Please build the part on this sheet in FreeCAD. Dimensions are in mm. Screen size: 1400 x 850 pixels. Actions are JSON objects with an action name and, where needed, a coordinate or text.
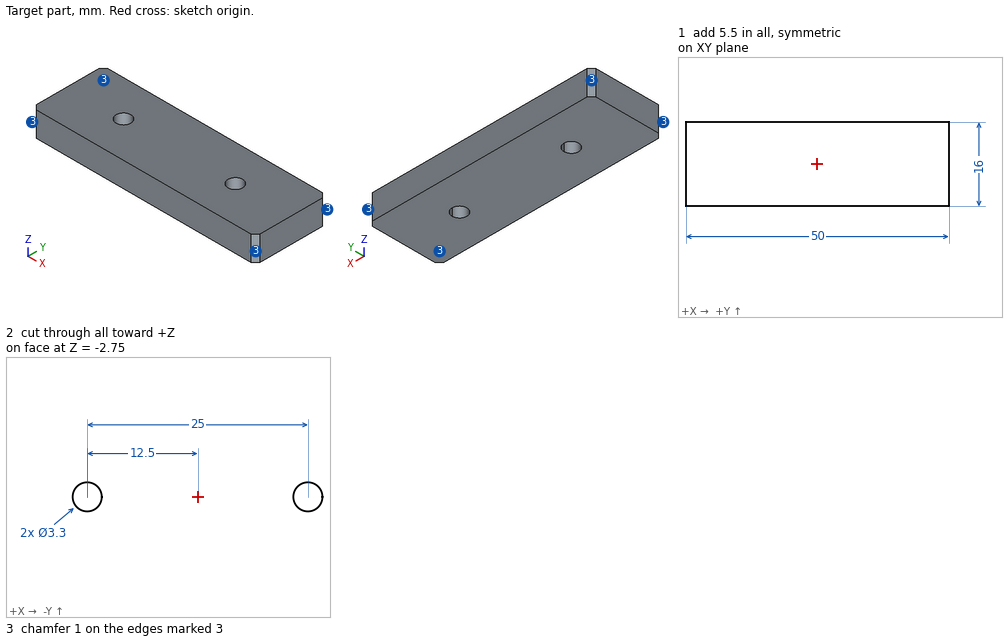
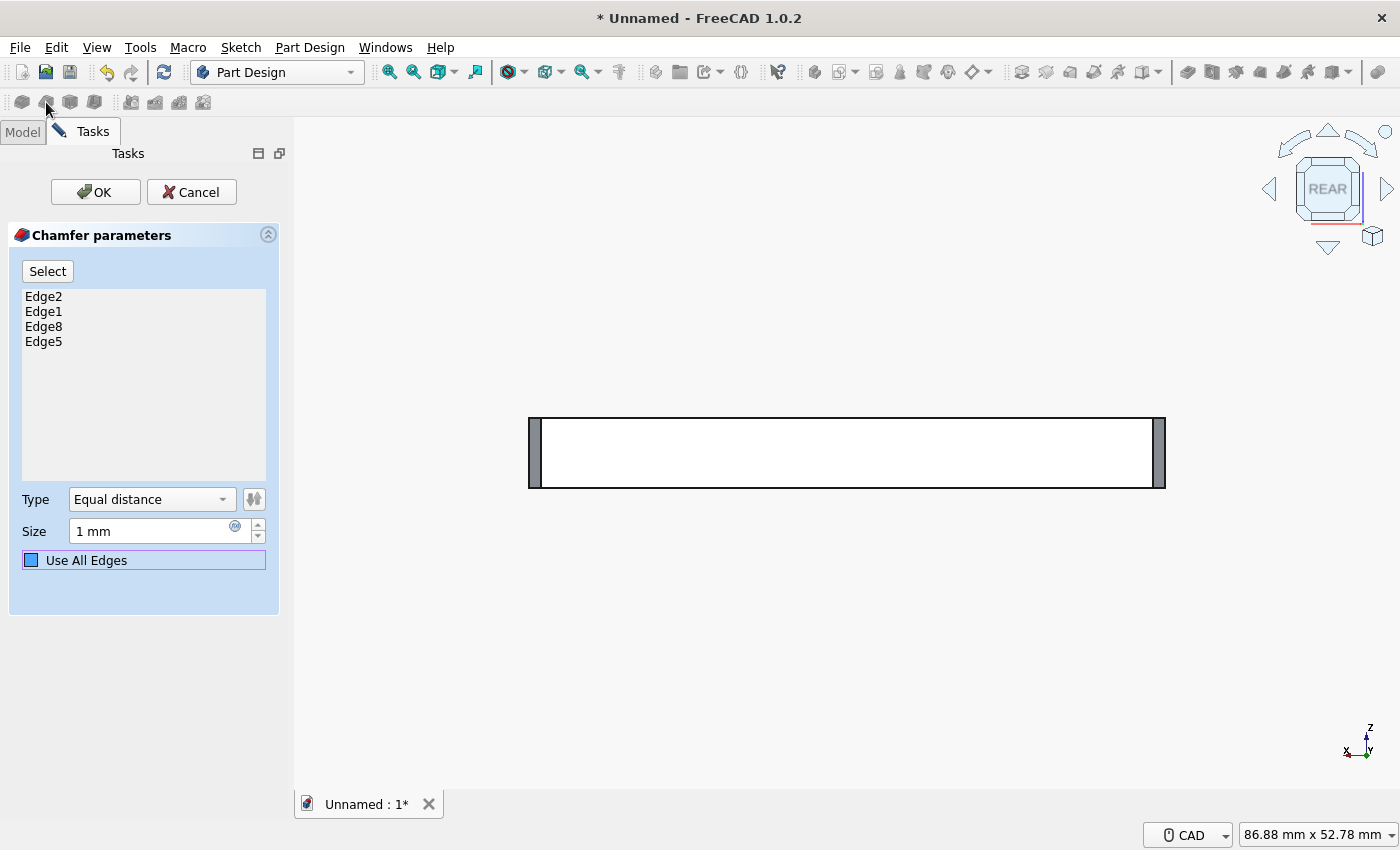
{"action": "left_click", "coordinate": [96, 192]}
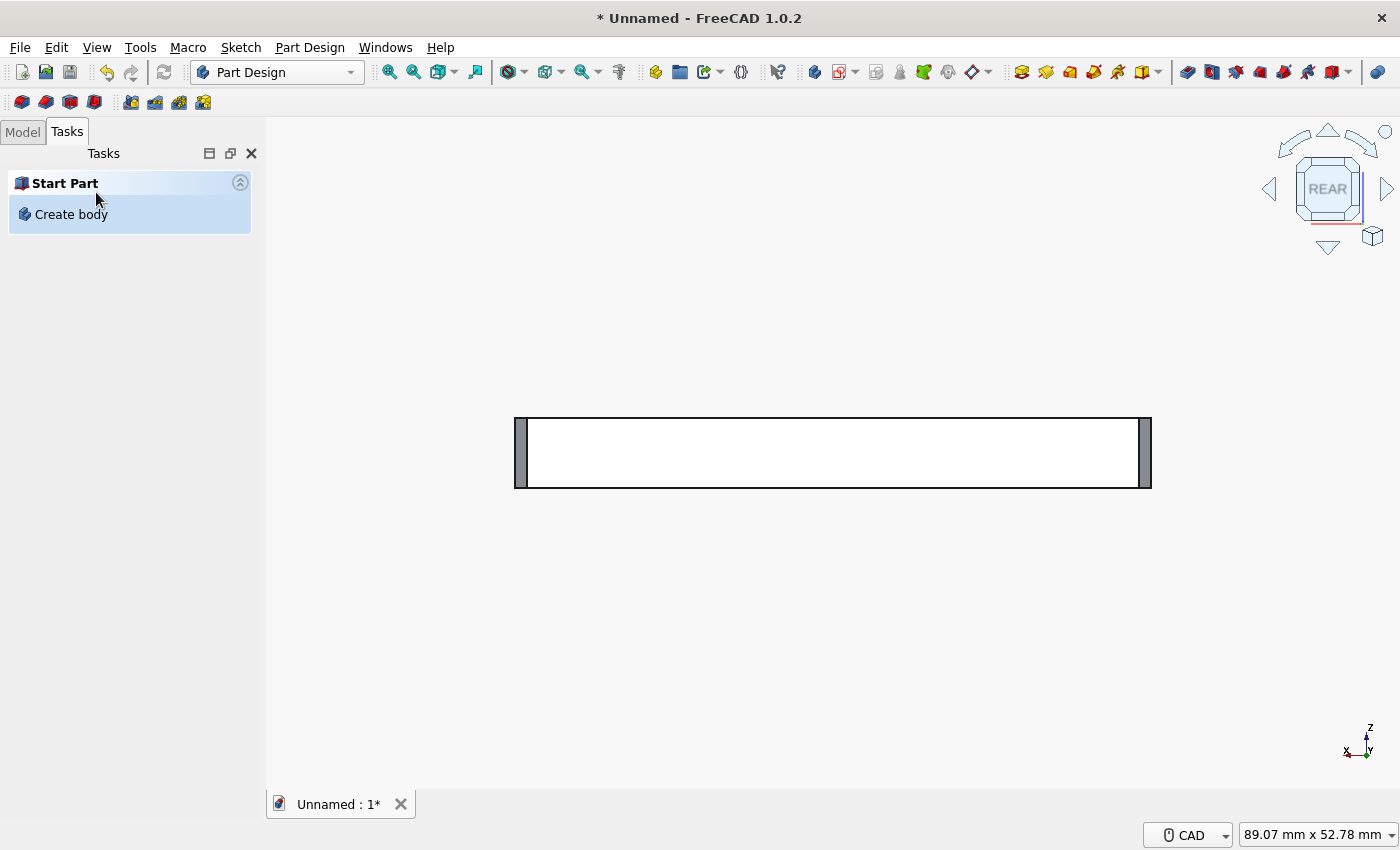
{"action": "key", "text": "0"}